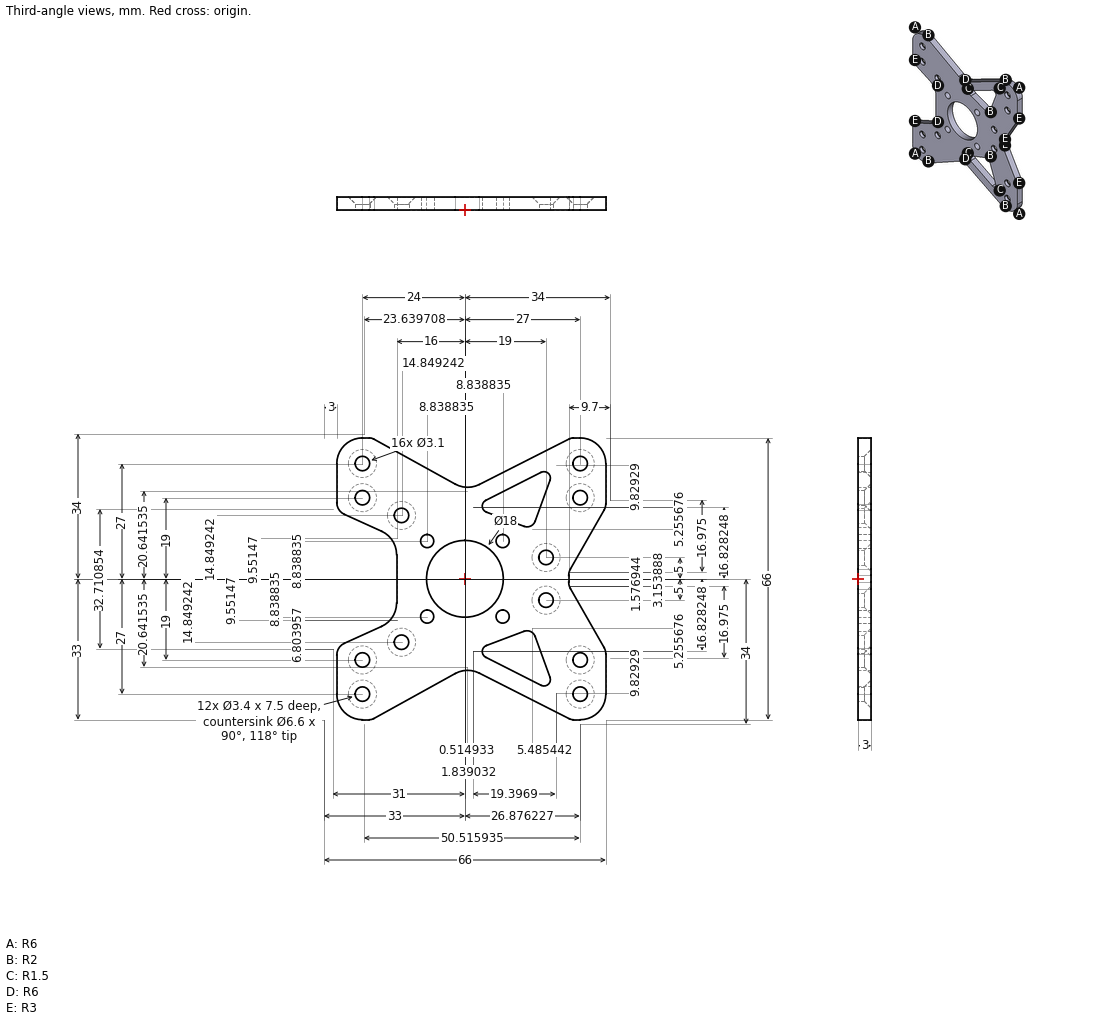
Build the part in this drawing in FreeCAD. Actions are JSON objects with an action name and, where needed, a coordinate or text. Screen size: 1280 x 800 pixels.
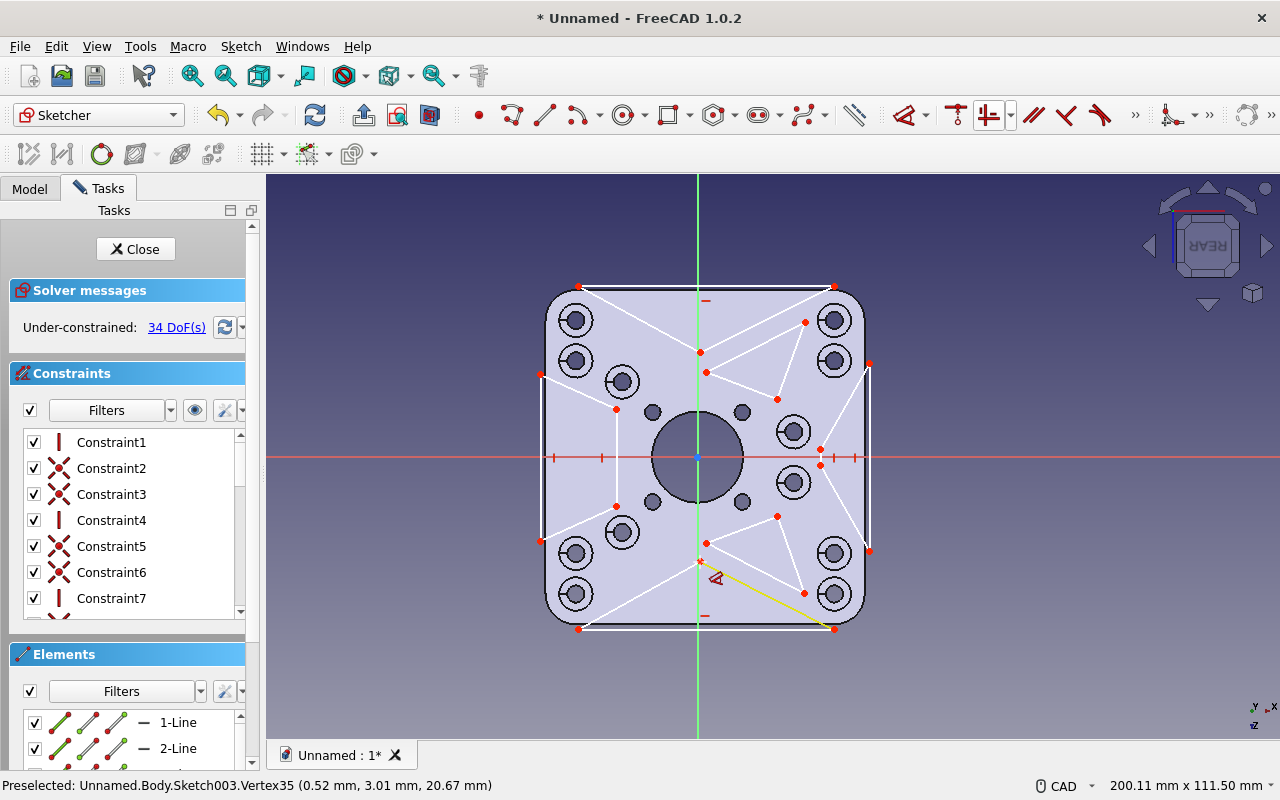
{"action": "left_click", "coordinate": [617, 507]}
{"action": "left_click", "coordinate": [657, 541]}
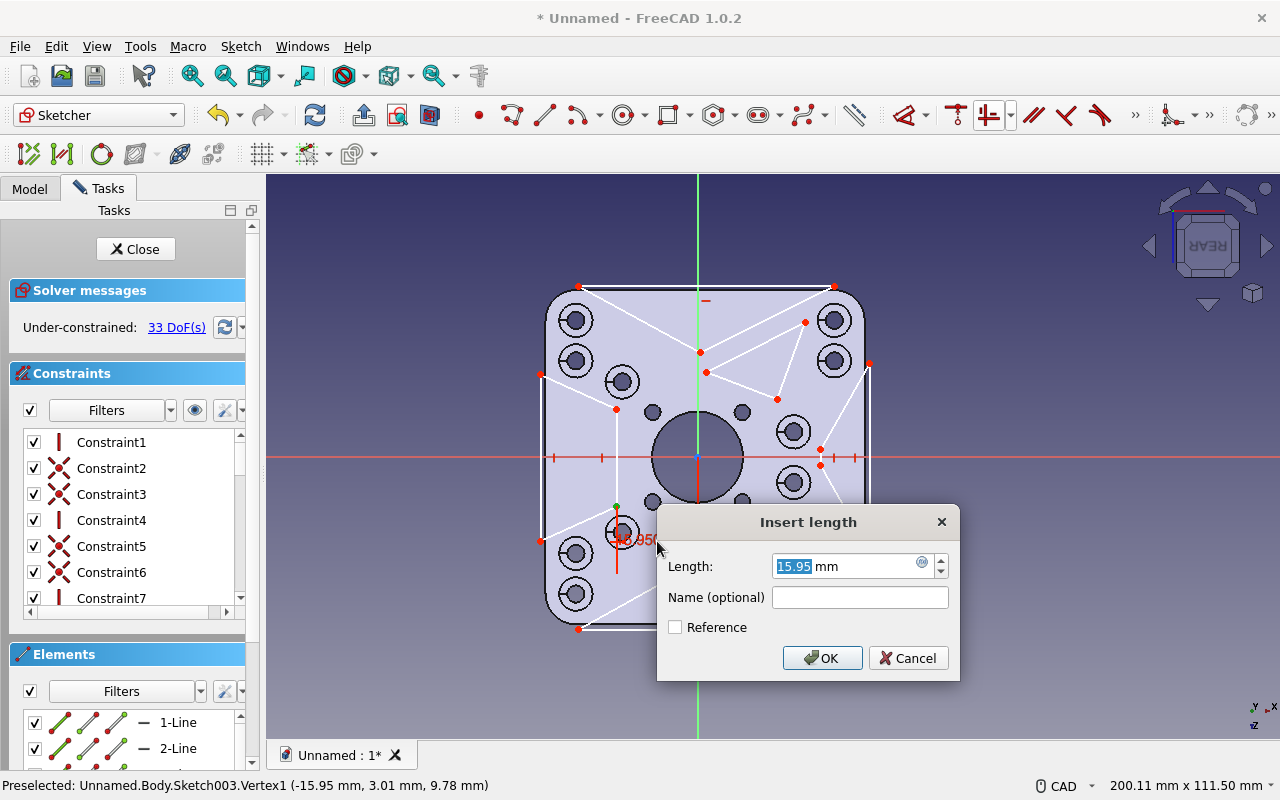
{"action": "type", "text": "16"}
{"action": "key", "text": "Return"}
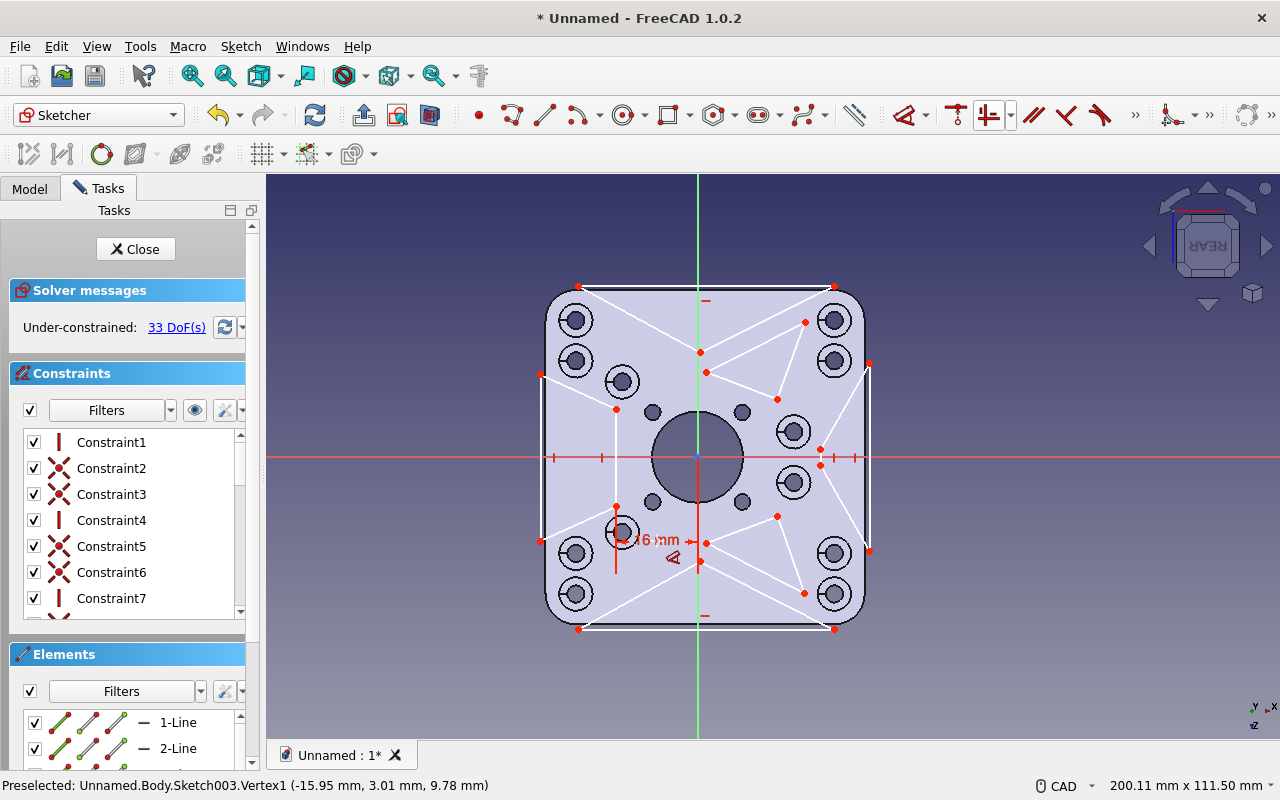
{"action": "left_click", "coordinate": [541, 375]}
{"action": "left_click", "coordinate": [619, 341]}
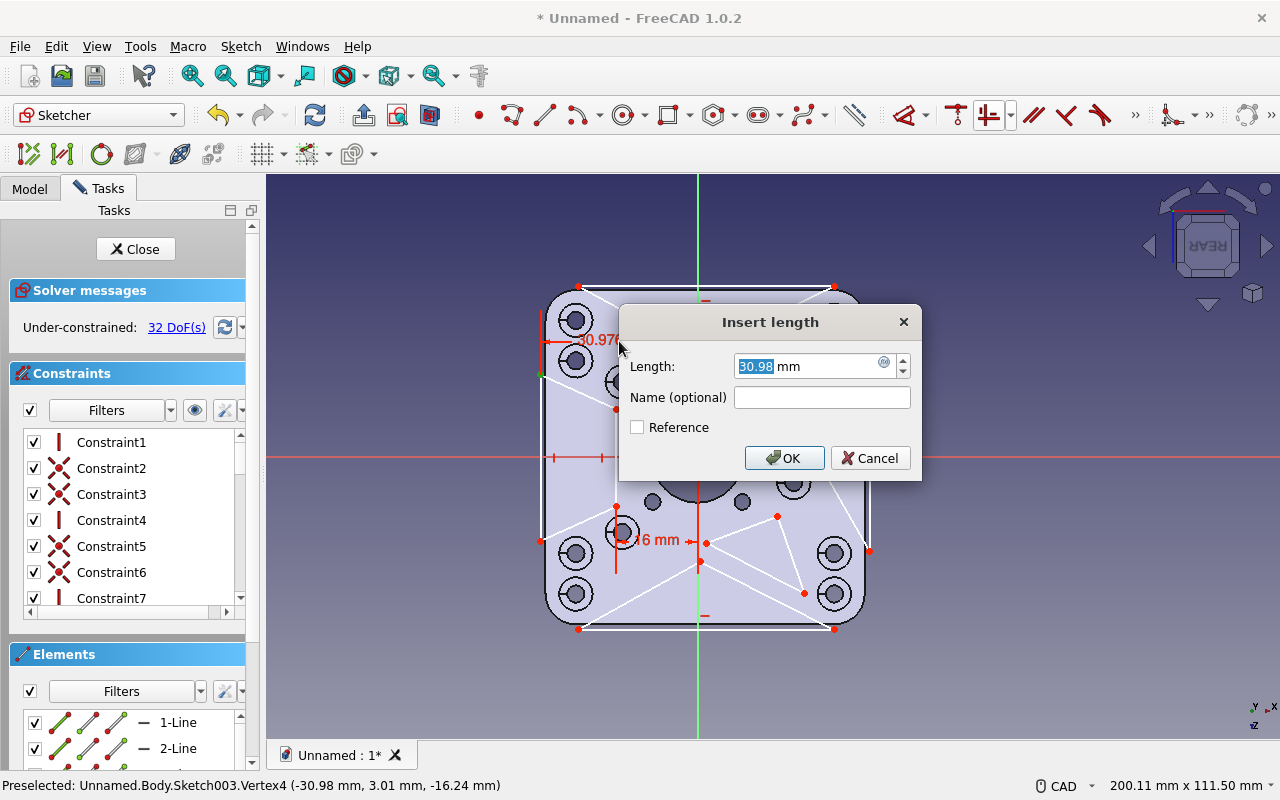
{"action": "type", "text": "31"}
{"action": "key", "text": "Return"}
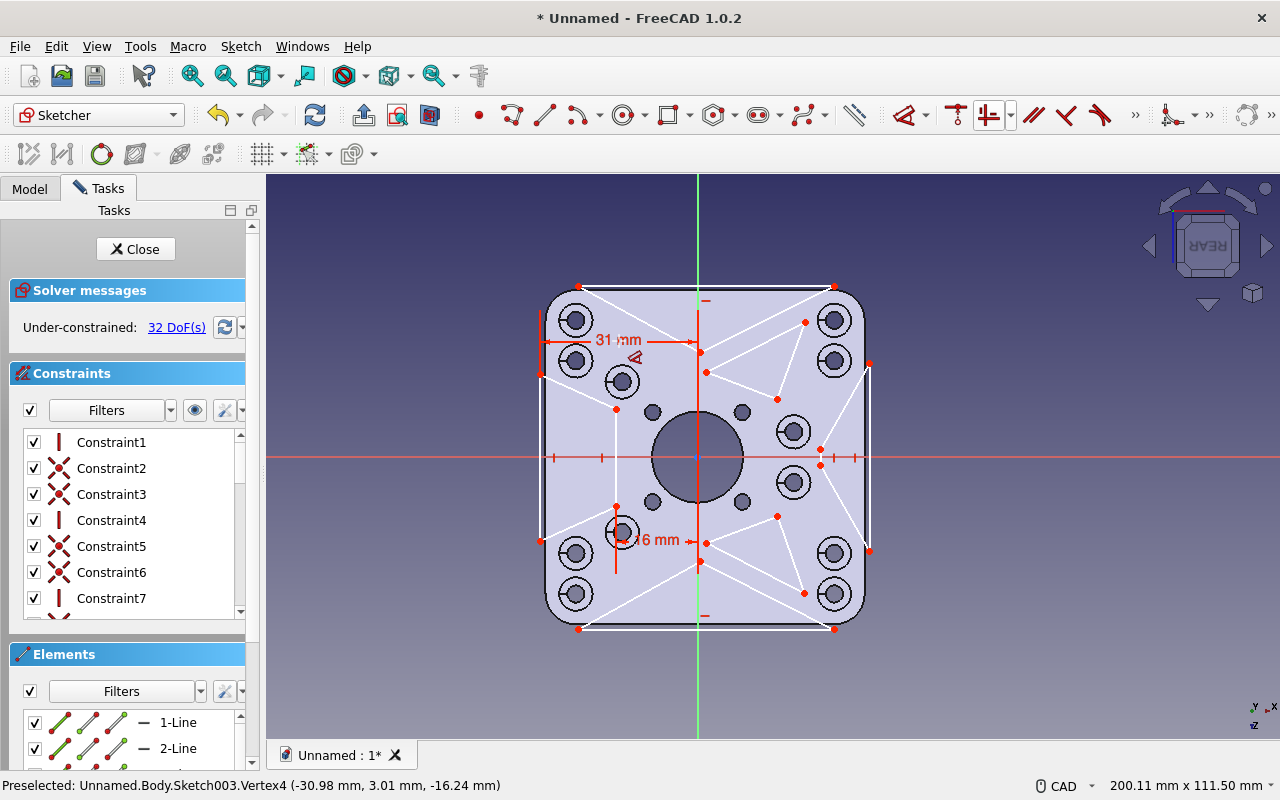
{"action": "left_click", "coordinate": [870, 552]}
{"action": "left_click", "coordinate": [823, 586]}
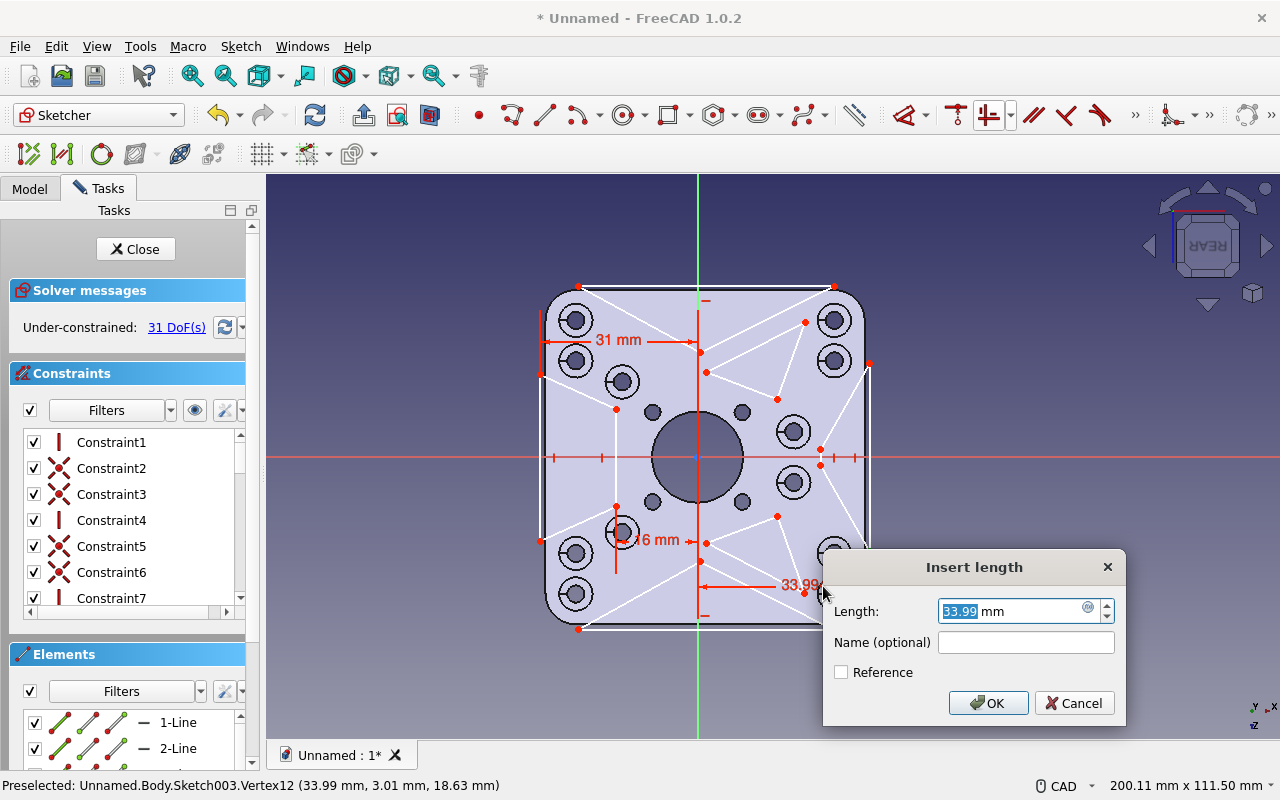
{"action": "type", "text": "34"}
{"action": "key", "text": "Return"}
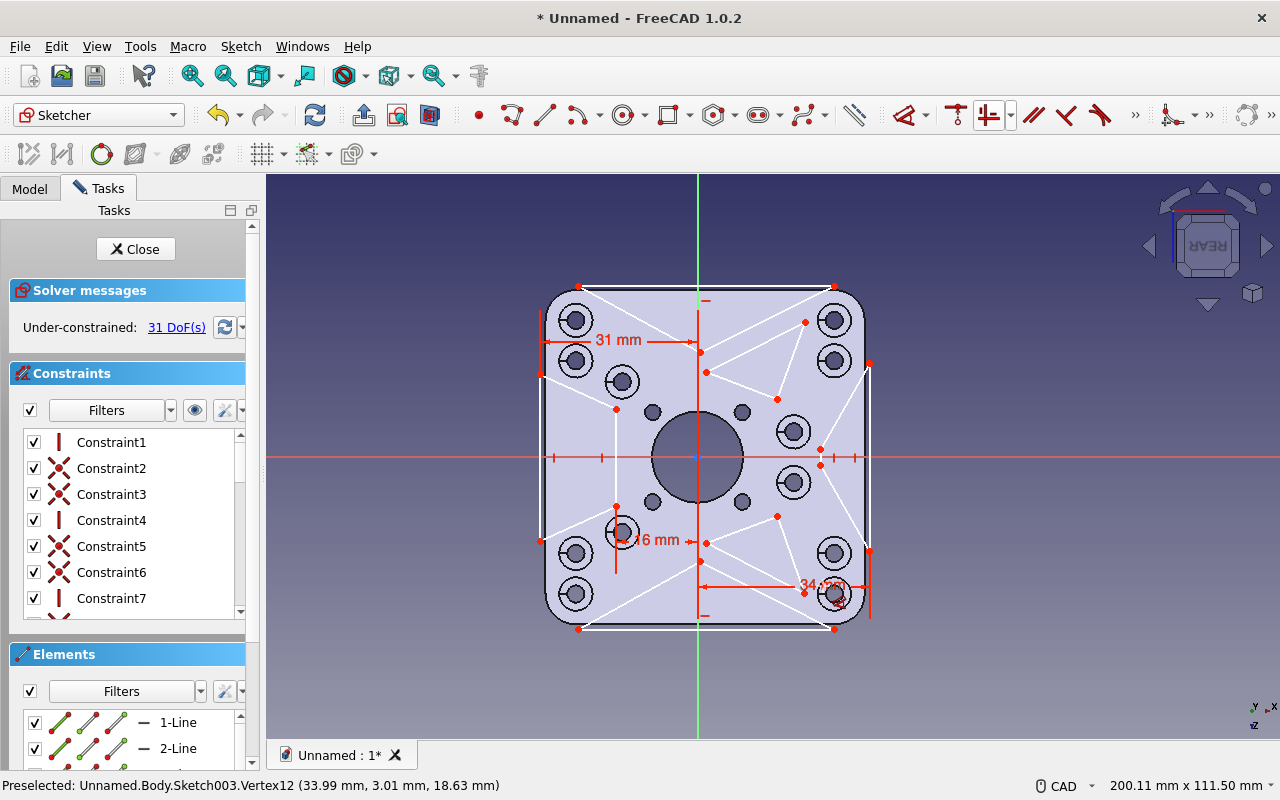
{"action": "left_click", "coordinate": [834, 286]}
{"action": "left_click", "coordinate": [868, 332]}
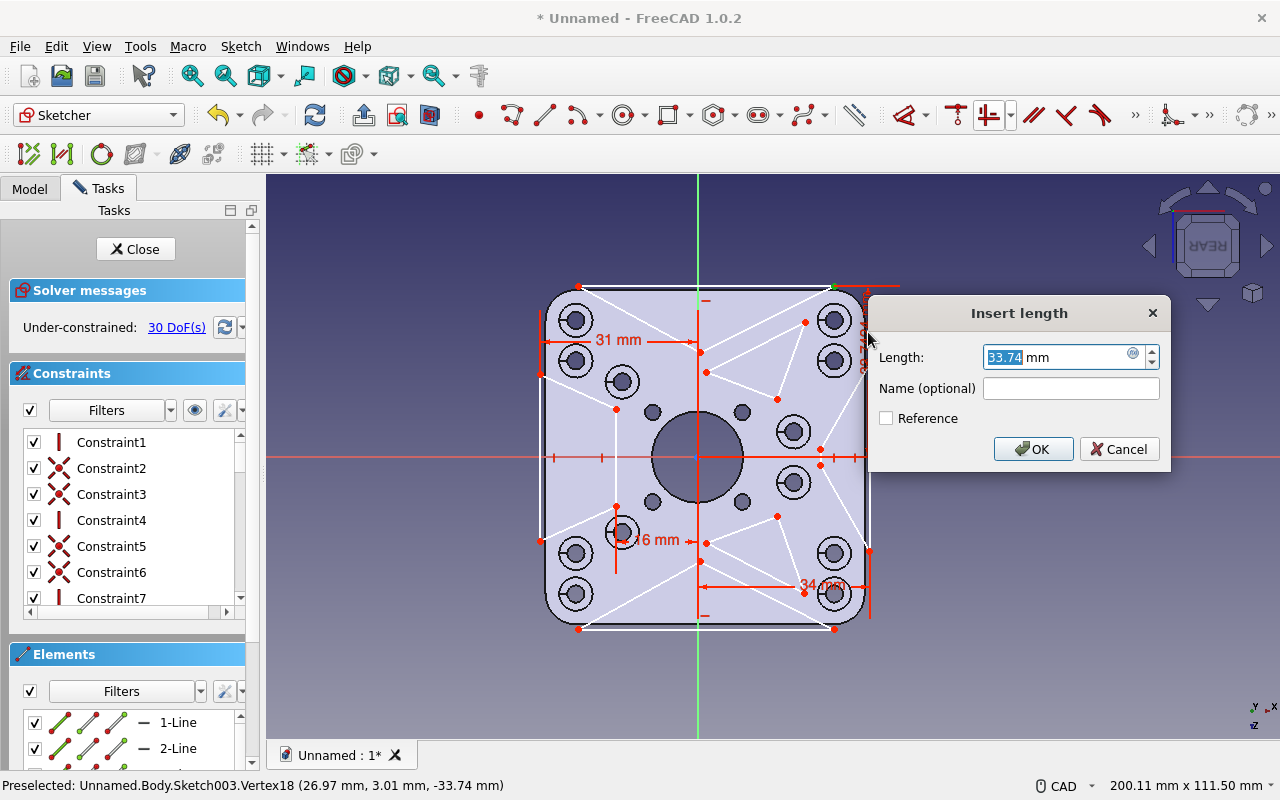
{"action": "type", "text": "34"}
{"action": "key", "text": "Return"}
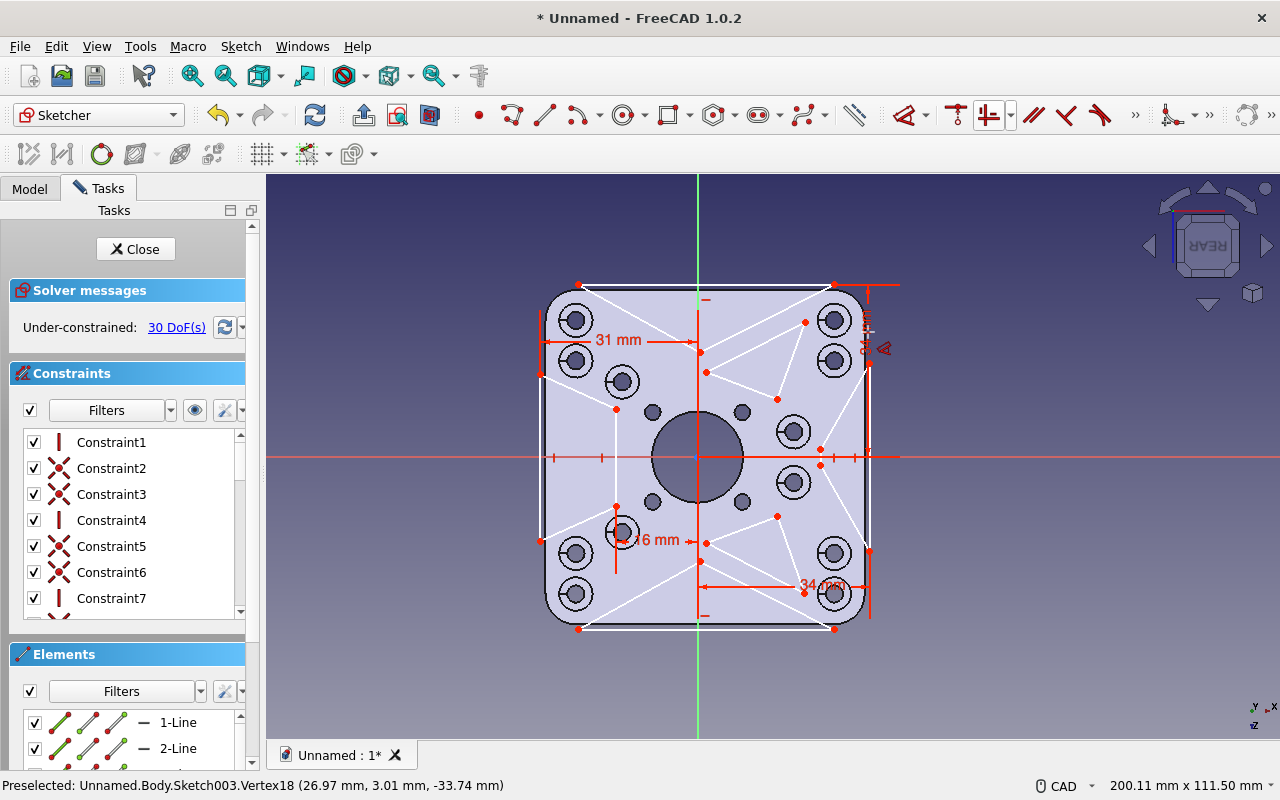
{"action": "left_click", "coordinate": [578, 630]}
{"action": "left_click", "coordinate": [544, 583]}